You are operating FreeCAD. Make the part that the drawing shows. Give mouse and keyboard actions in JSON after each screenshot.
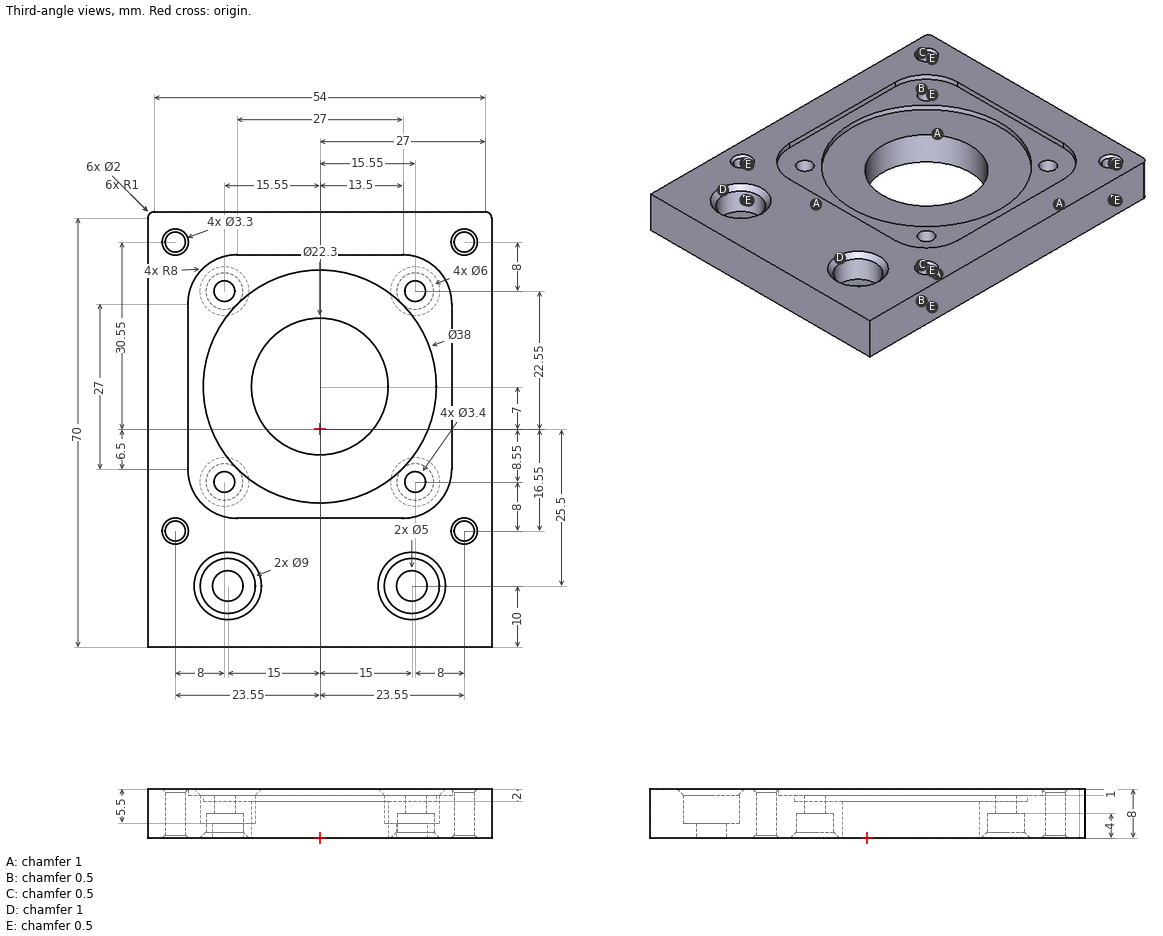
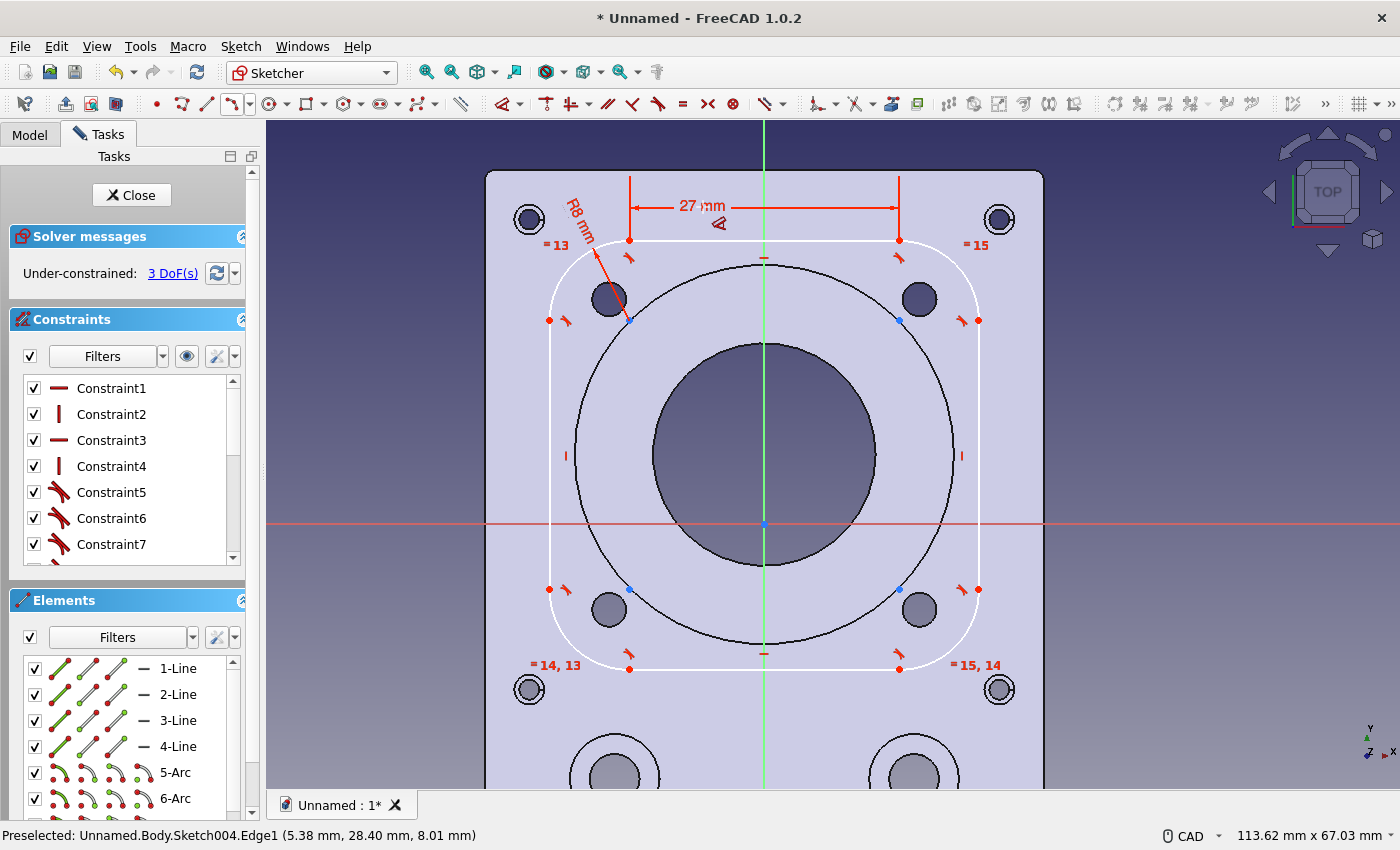
{"action": "left_click", "coordinate": [550, 402]}
{"action": "left_click", "coordinate": [516, 455]}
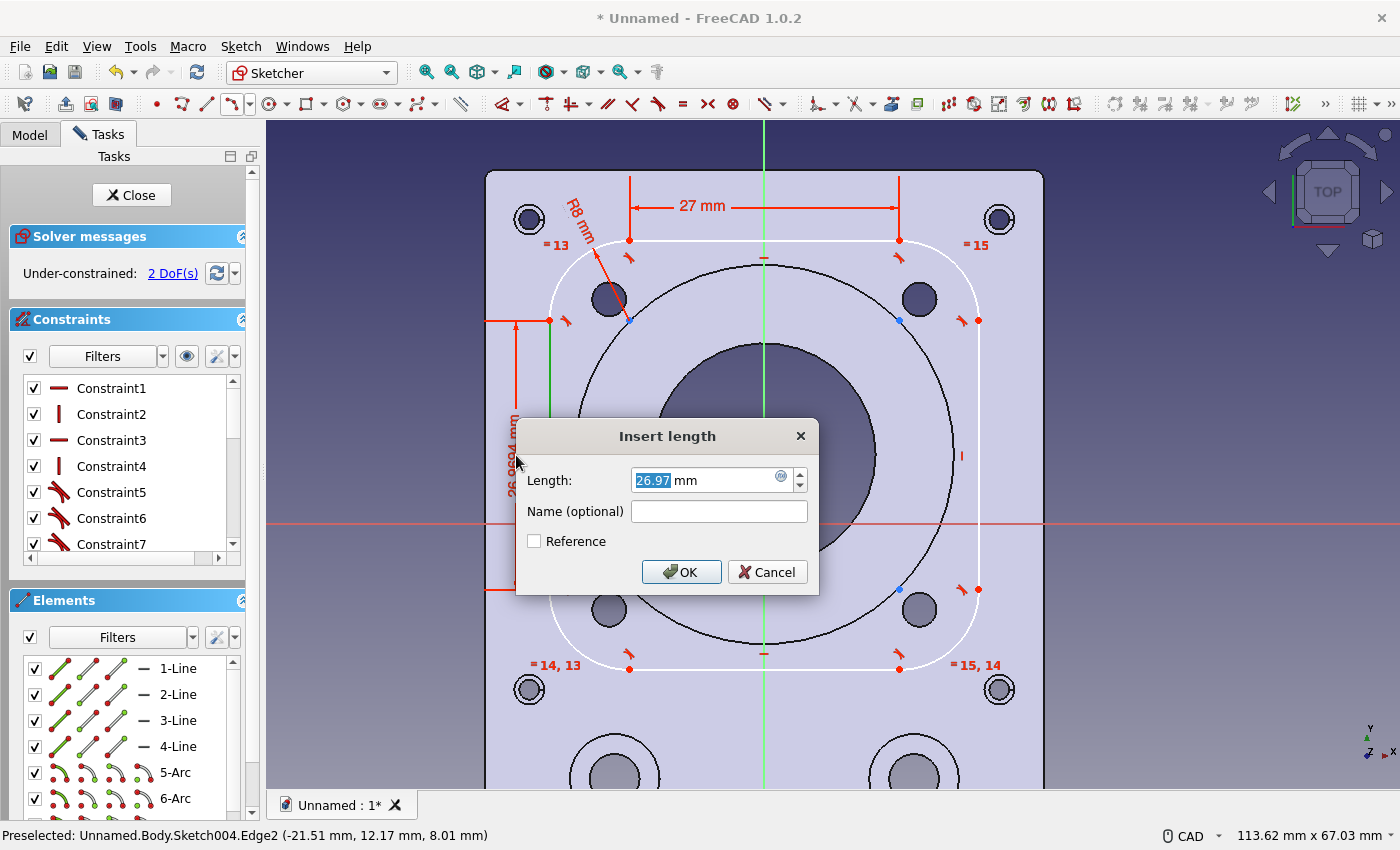
{"action": "type", "text": "27"}
{"action": "key", "text": "Return"}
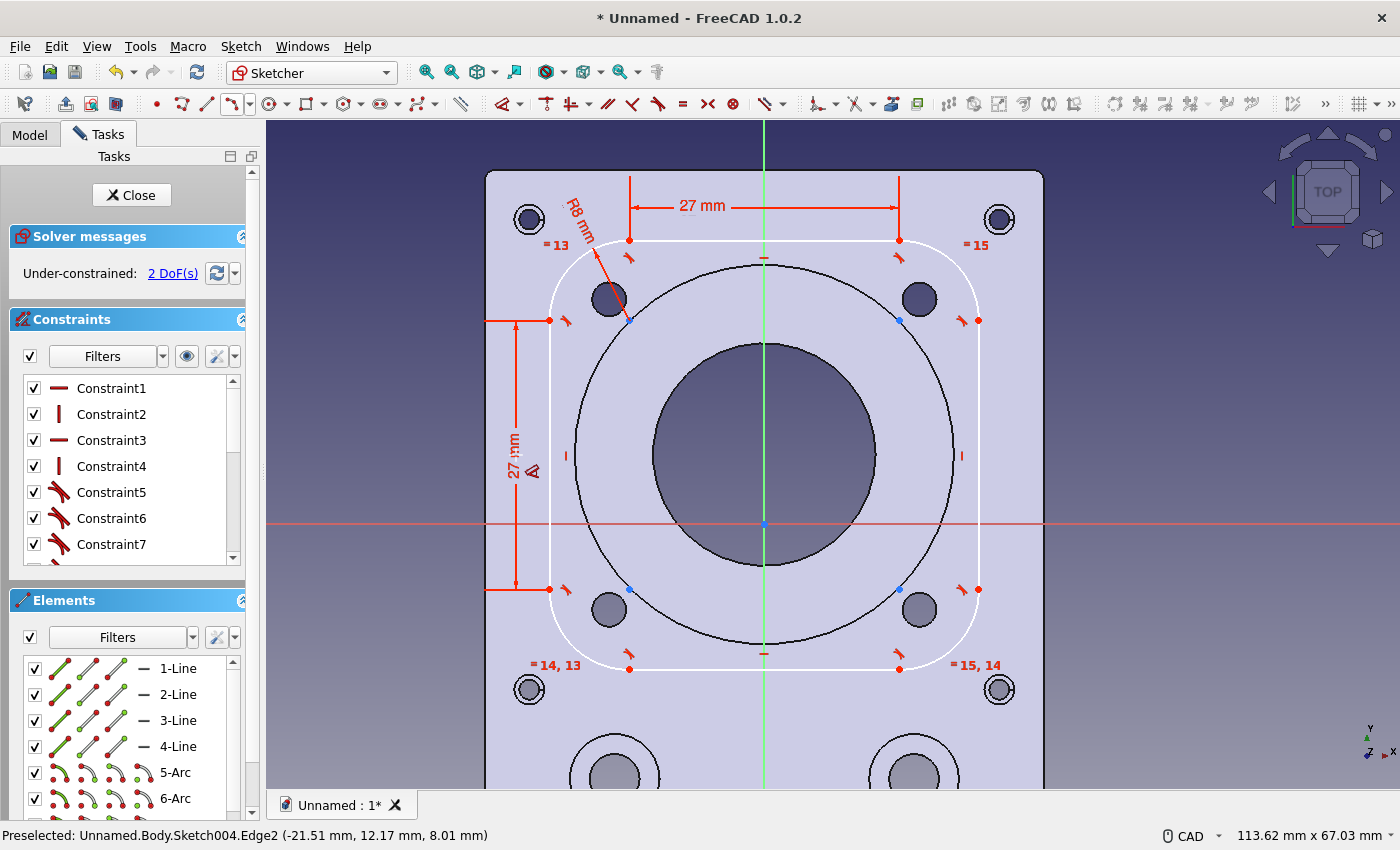
{"action": "left_click", "coordinate": [550, 590]}
{"action": "left_click", "coordinate": [516, 557]}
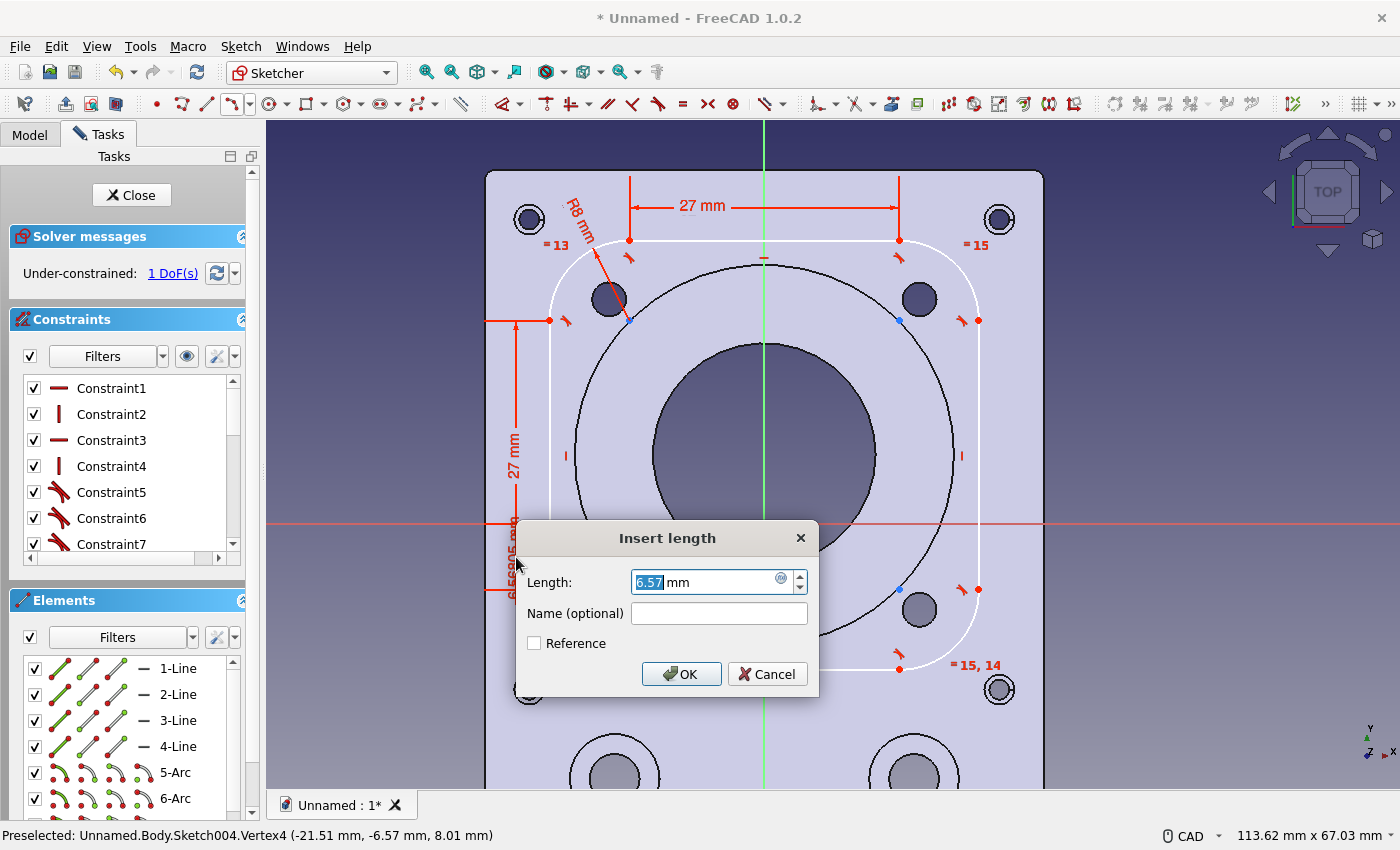
{"action": "type", "text": "6.5"}
{"action": "key", "text": "Return"}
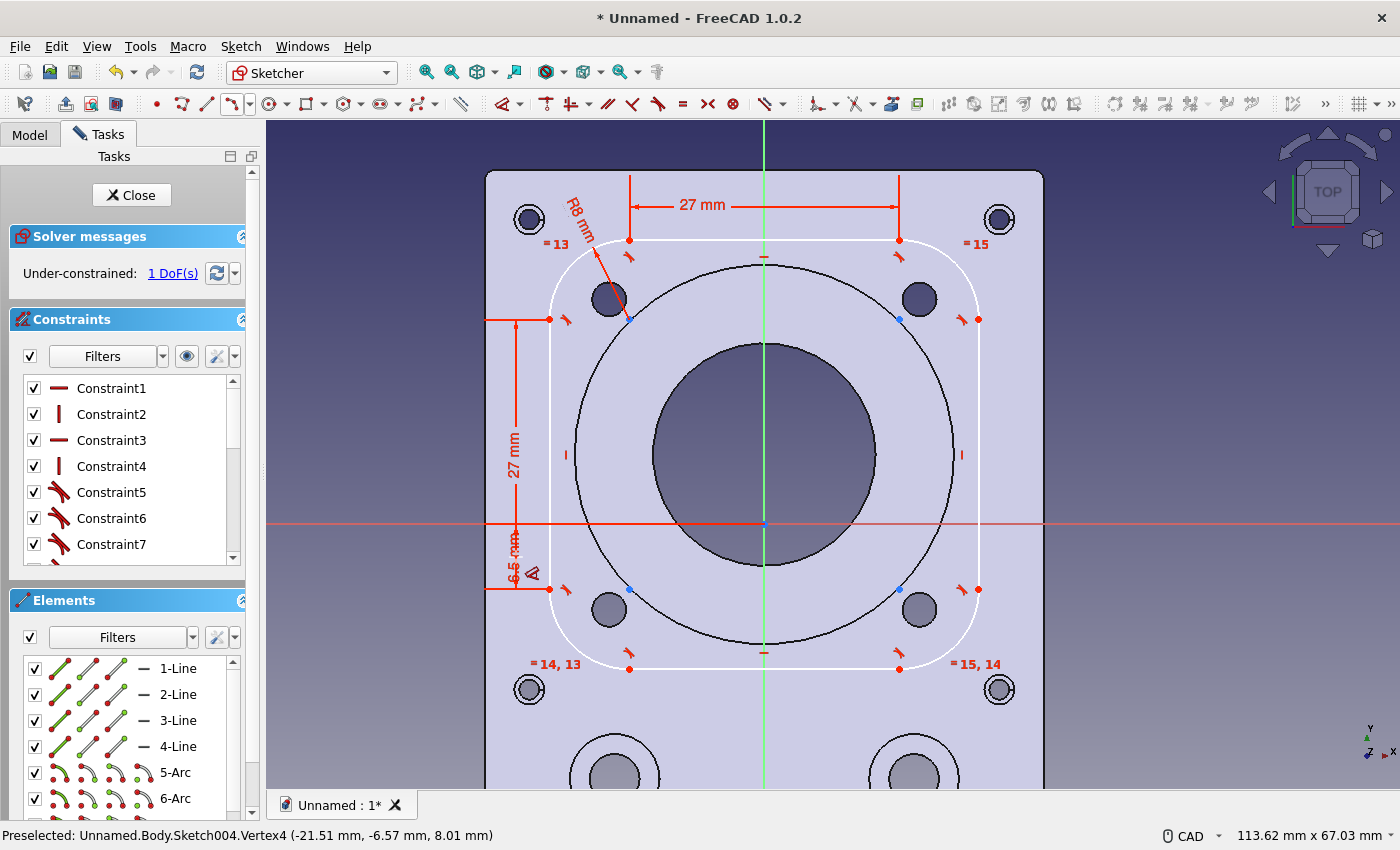
{"action": "left_click", "coordinate": [899, 240]}
{"action": "left_click", "coordinate": [832, 206]}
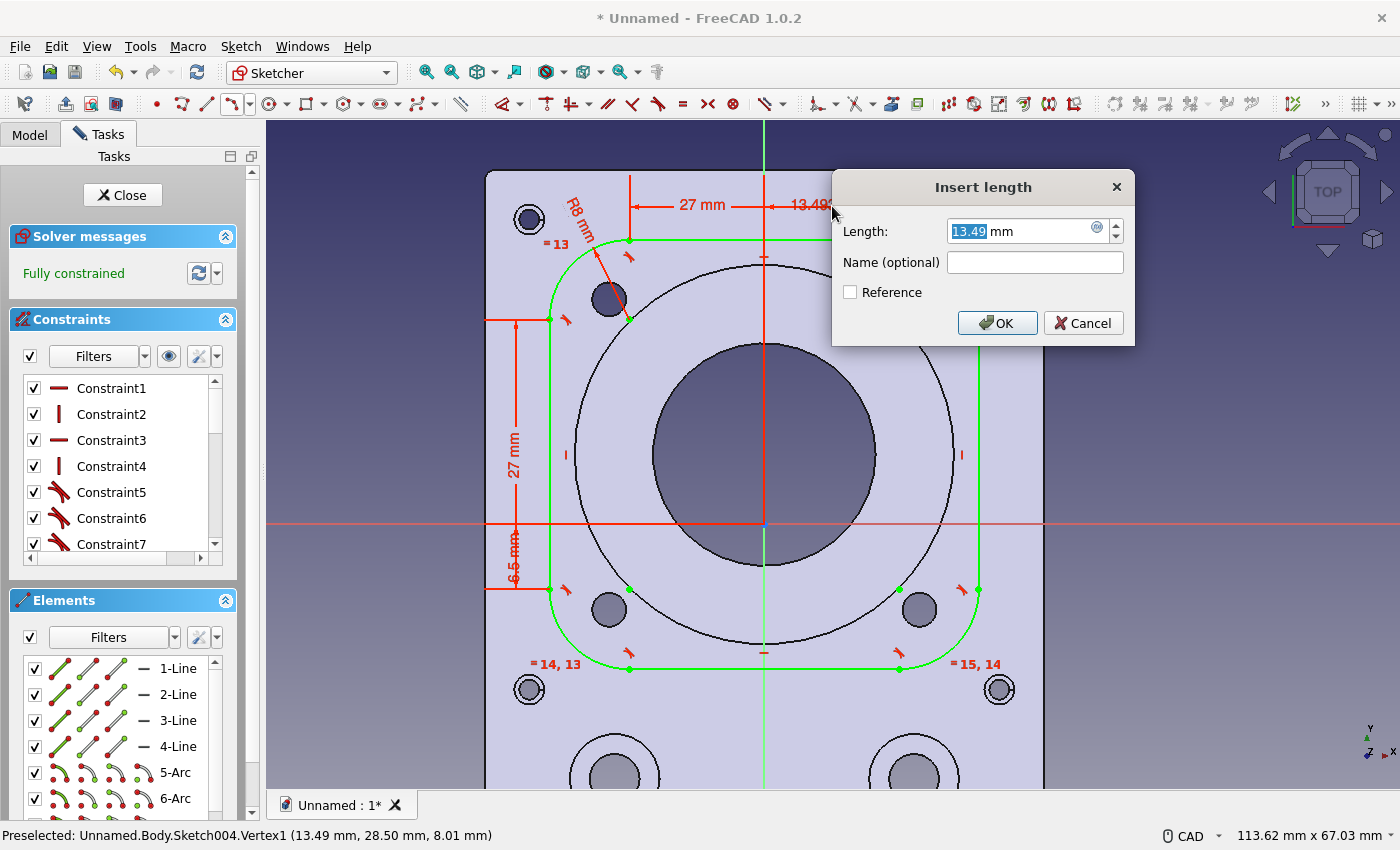
{"action": "type", "text": "13.5"}
{"action": "key", "text": "Return"}
{"action": "key", "text": "Escape"}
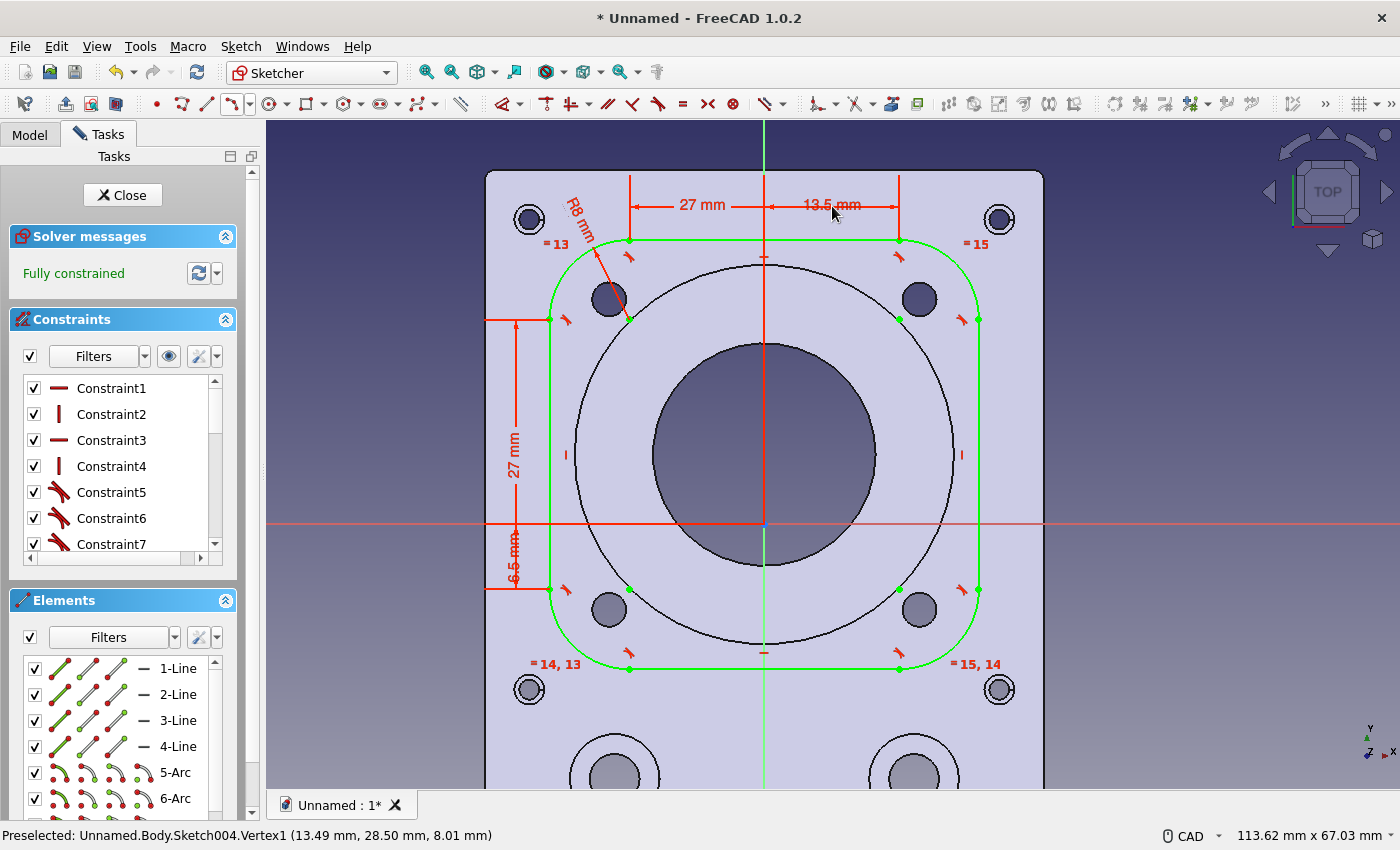
{"action": "left_click", "coordinate": [123, 195]}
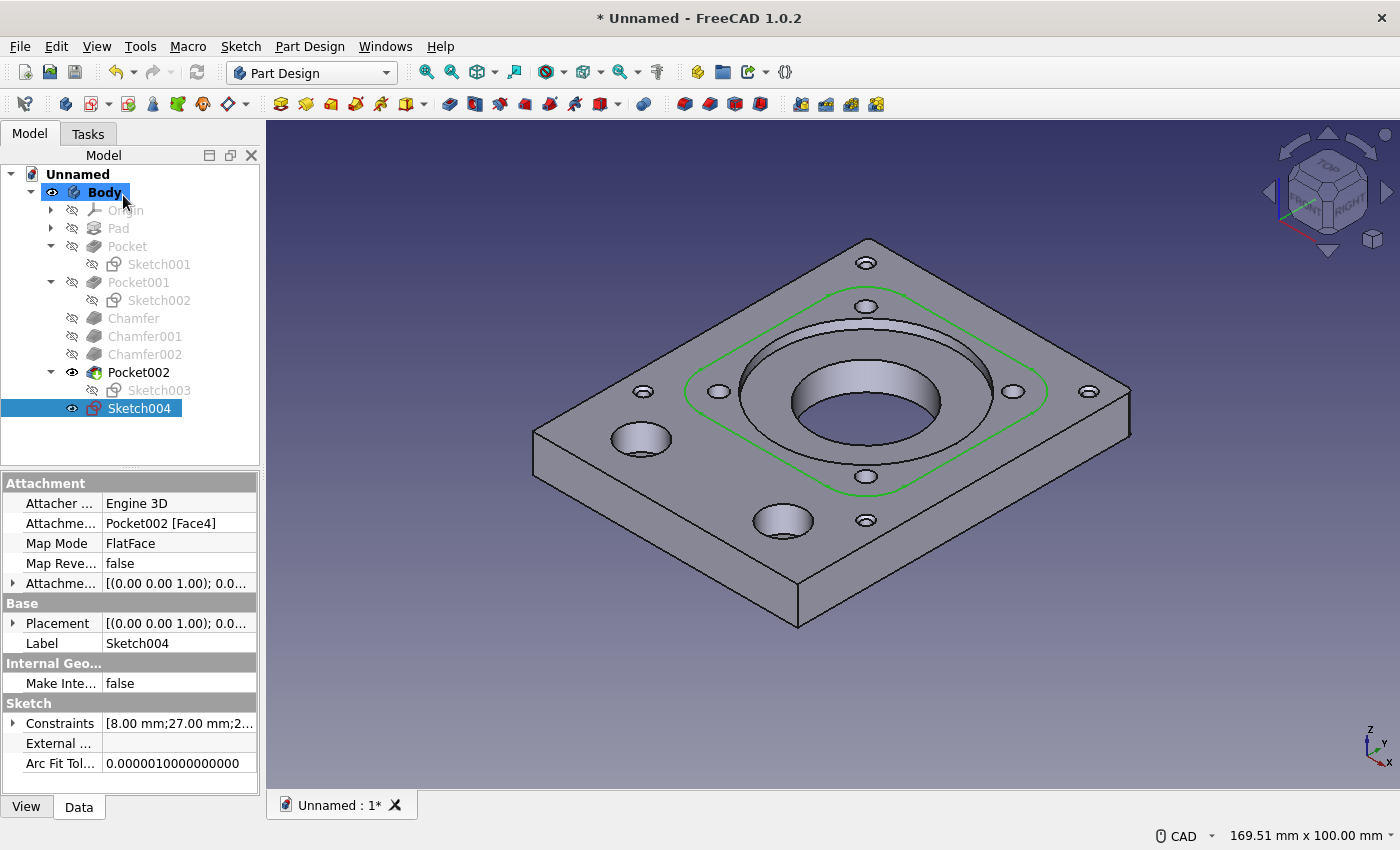
{"action": "left_click", "coordinate": [450, 104]}